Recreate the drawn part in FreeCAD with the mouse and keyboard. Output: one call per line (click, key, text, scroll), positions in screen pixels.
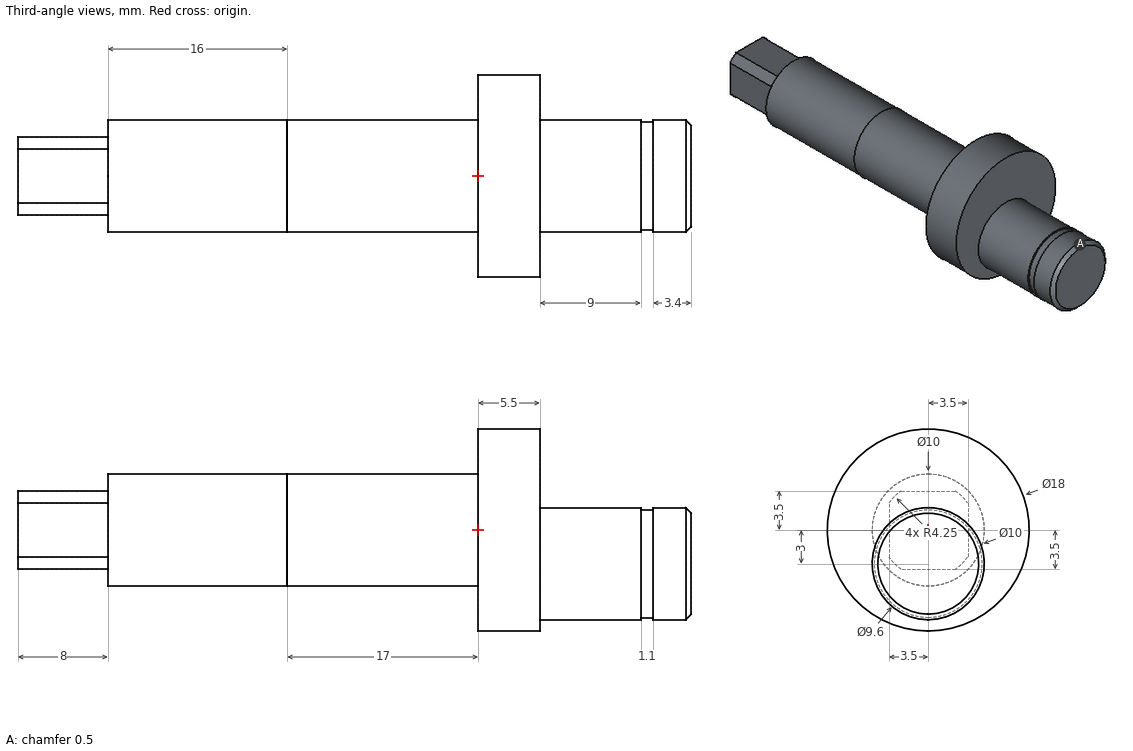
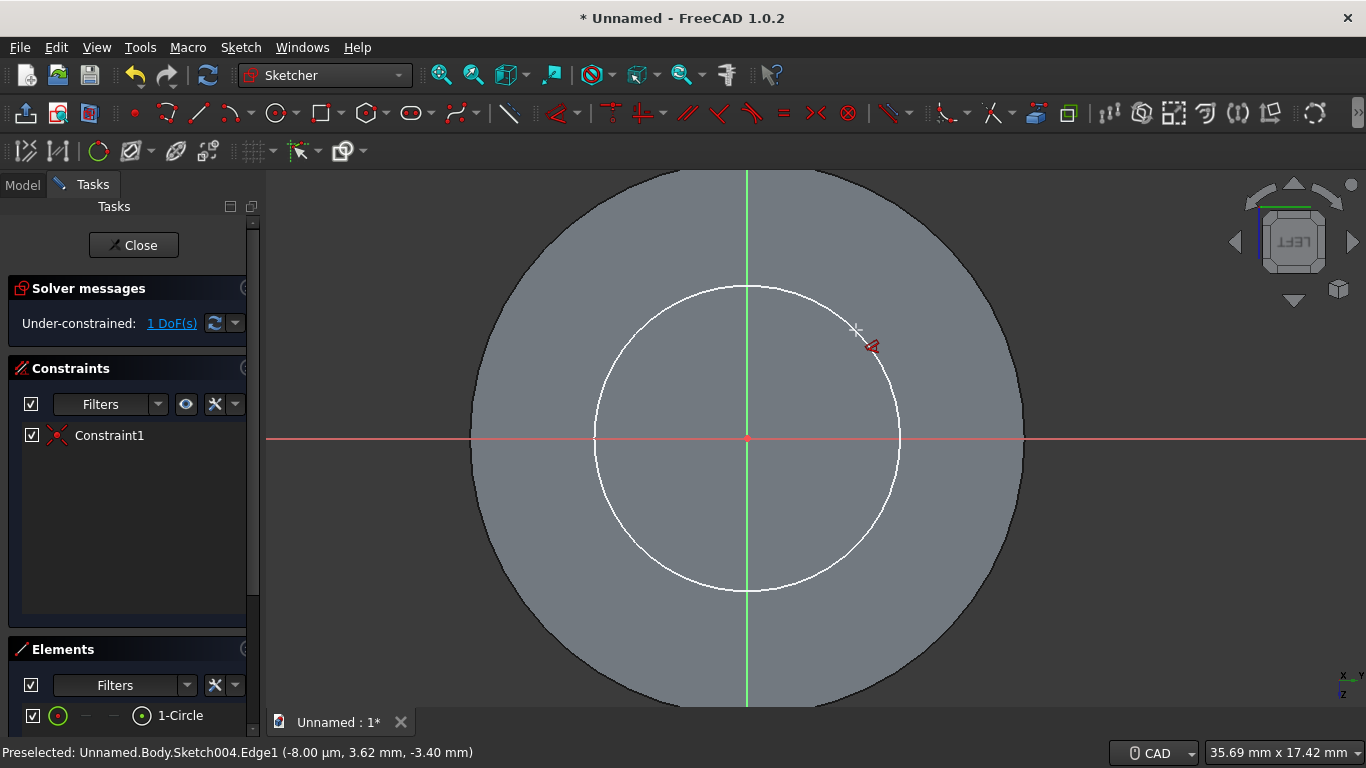
click(855, 330)
click(878, 307)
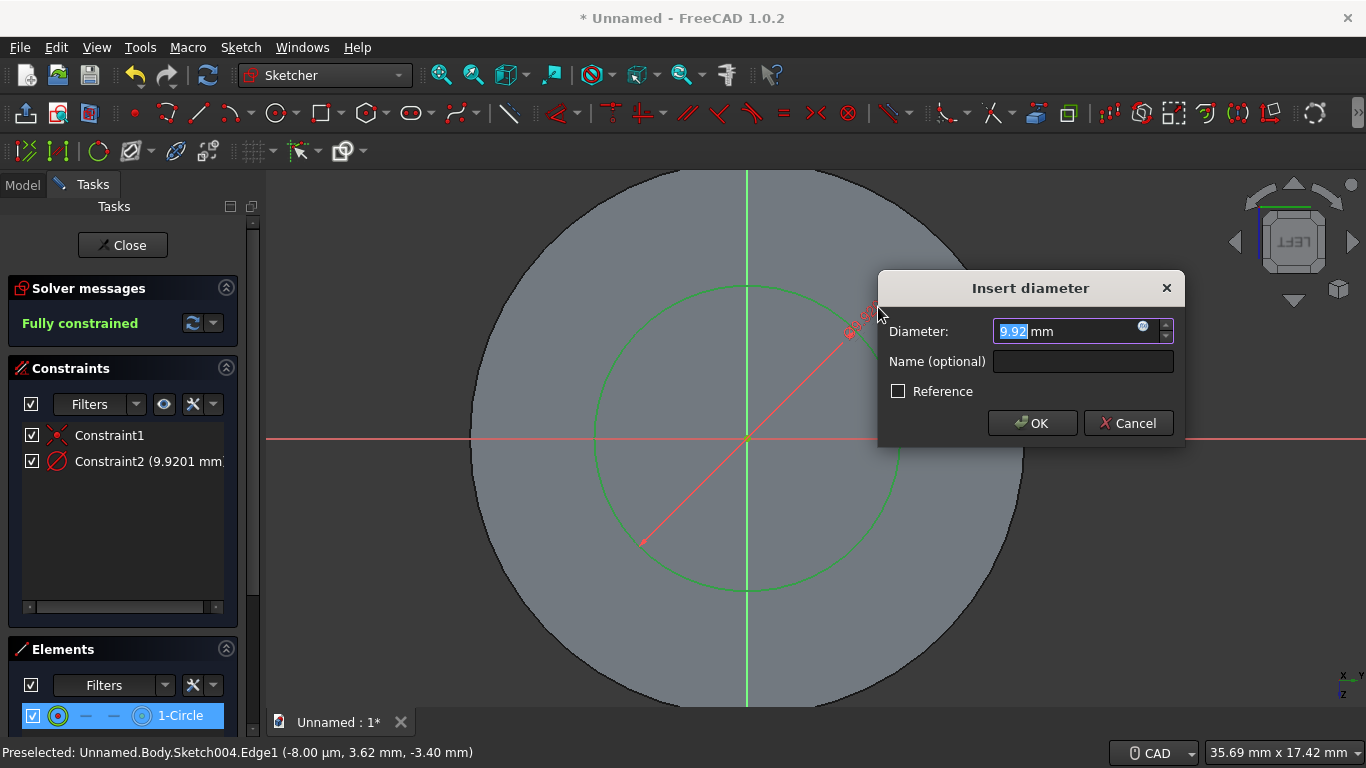
text(10)
key(Return)
key(Escape)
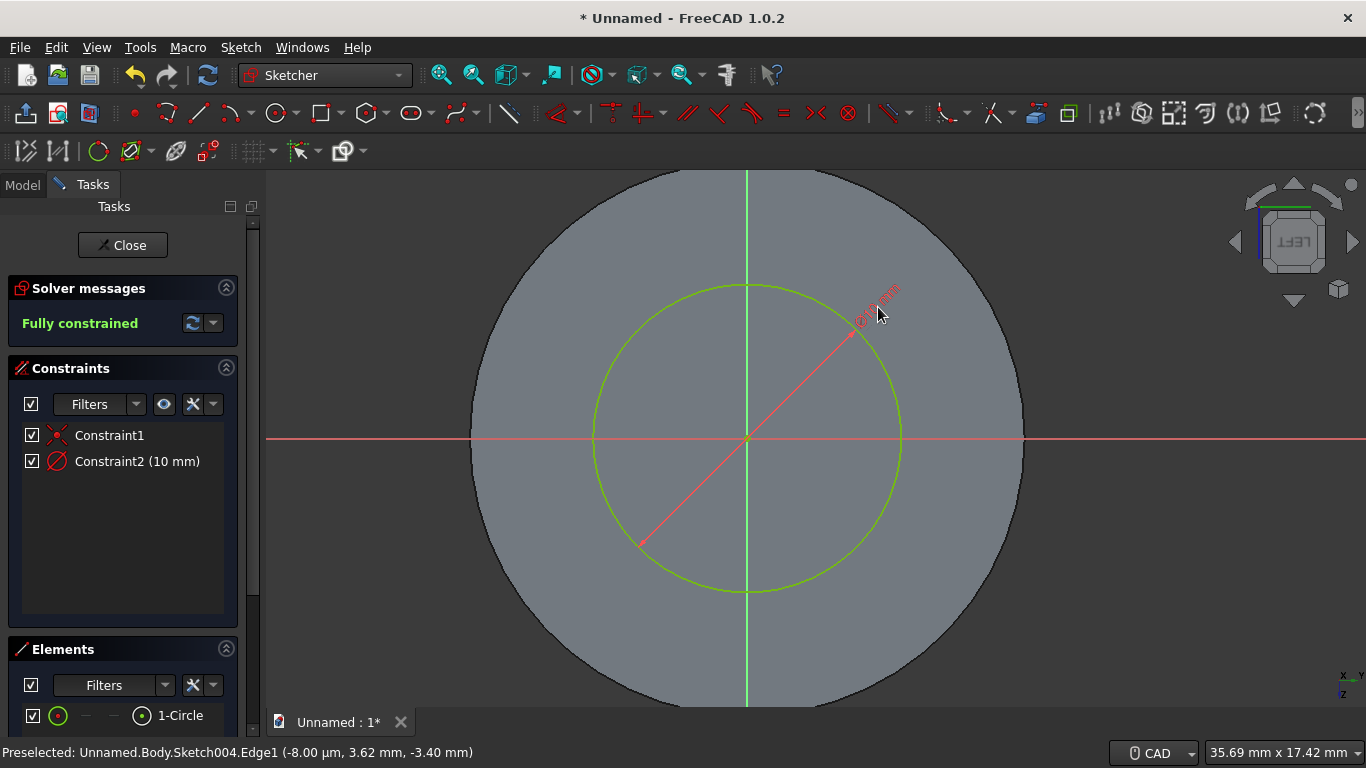
click(123, 245)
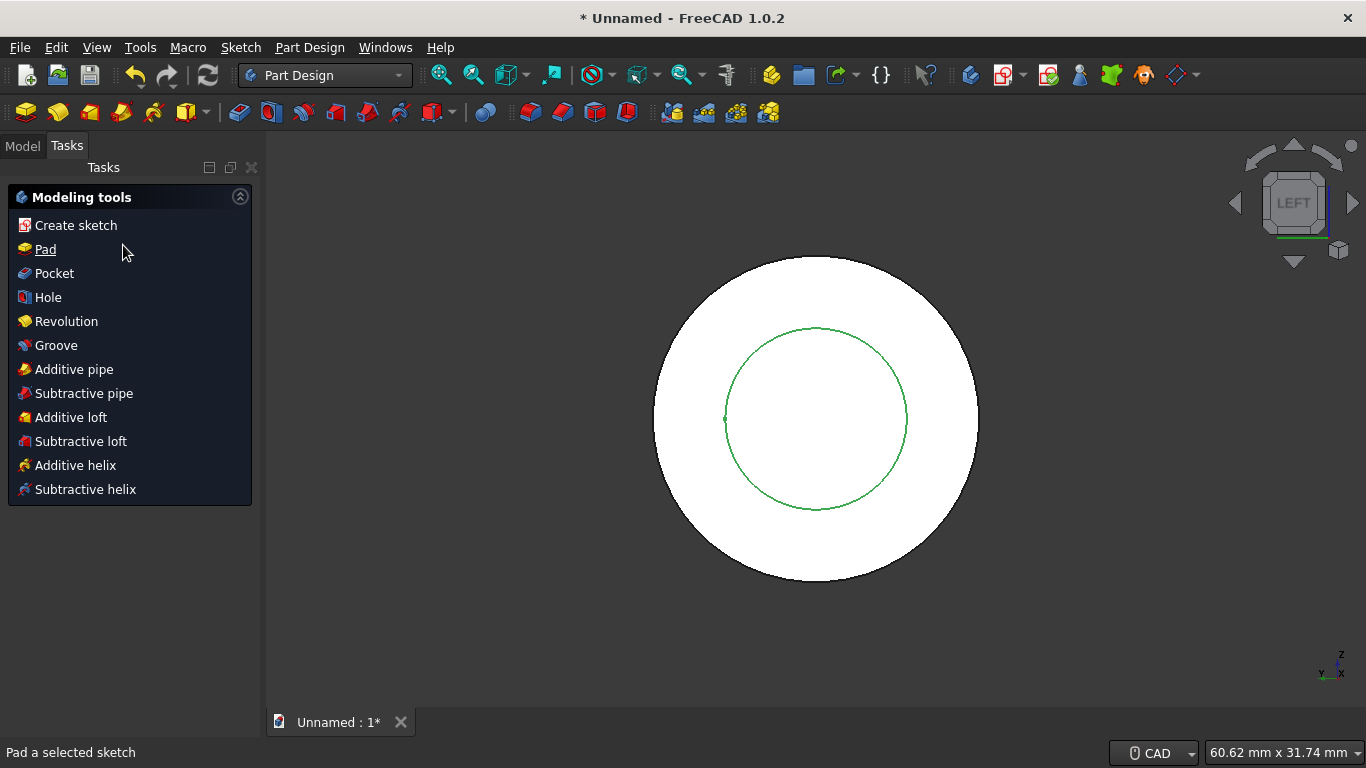
click(26, 112)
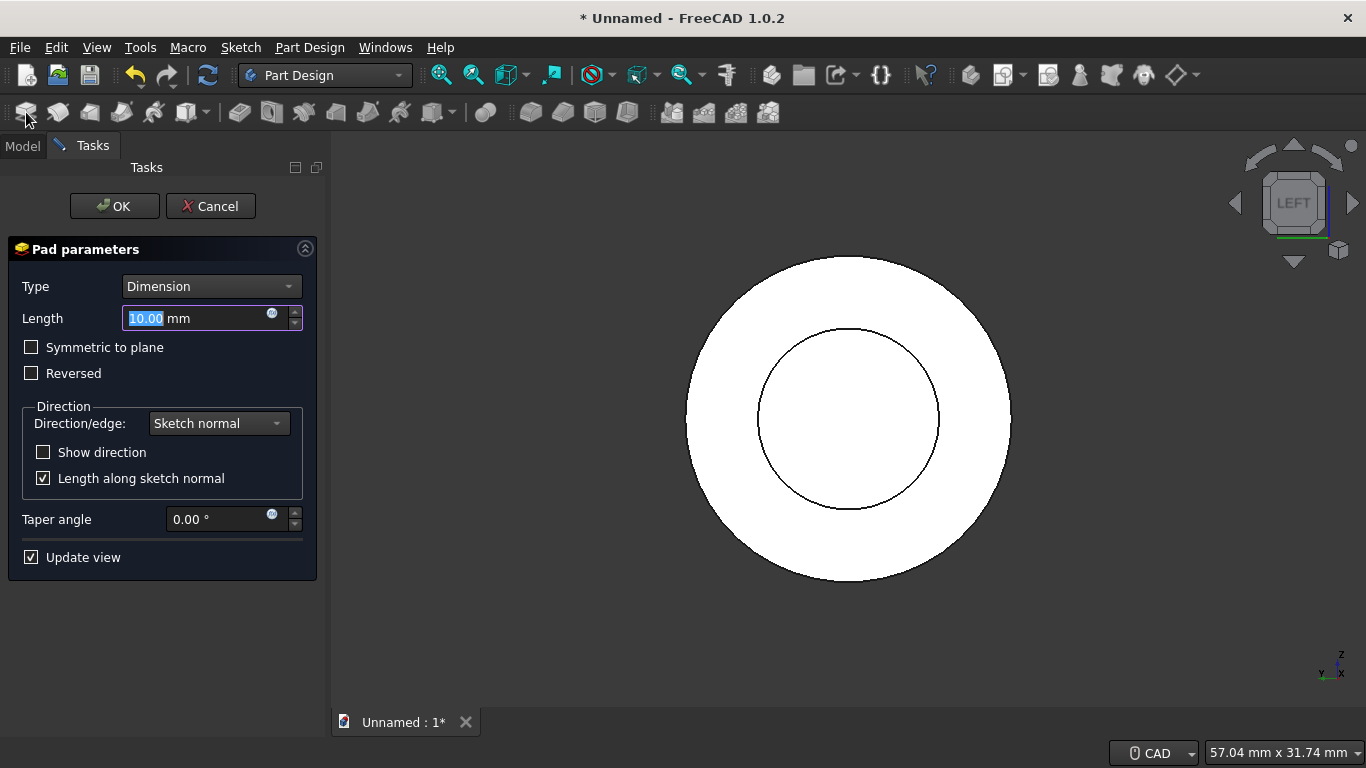
text(17)
key(Tab)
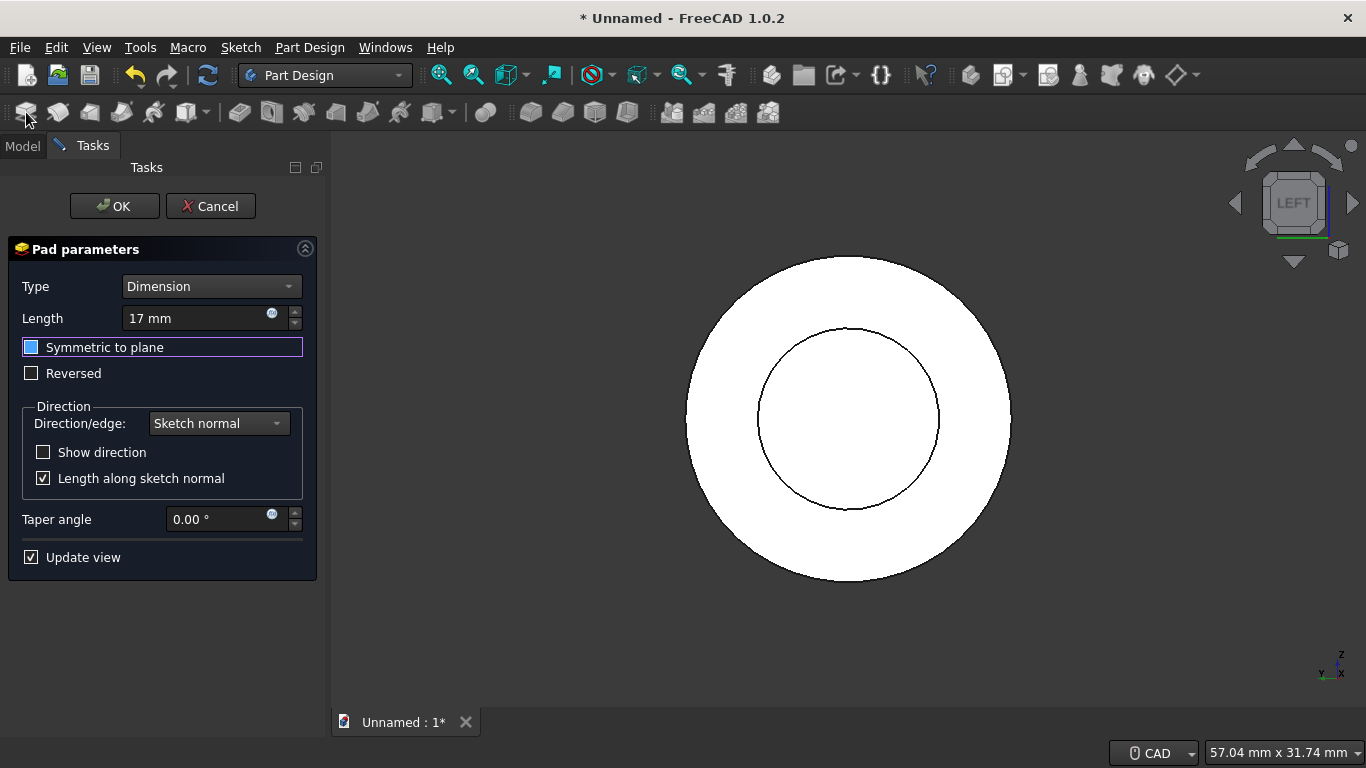
click(115, 206)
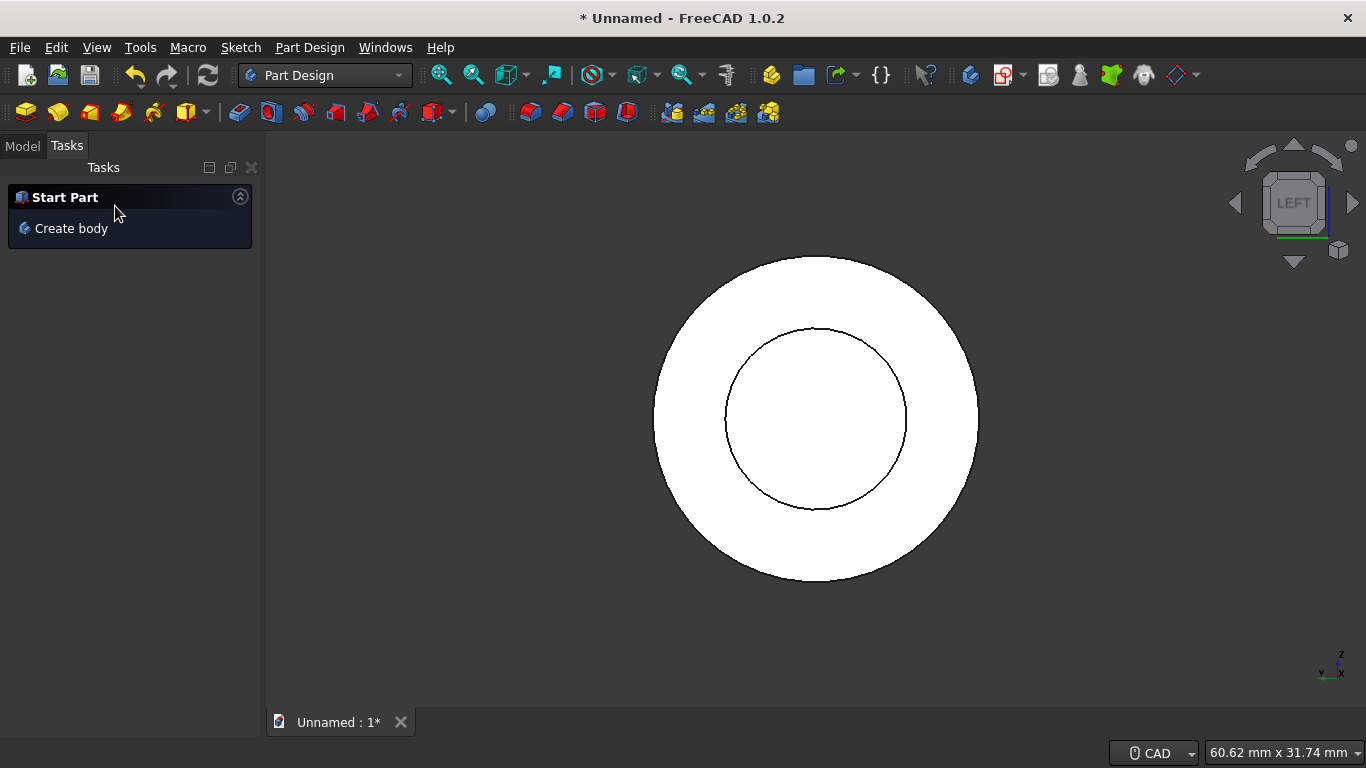
click(972, 76)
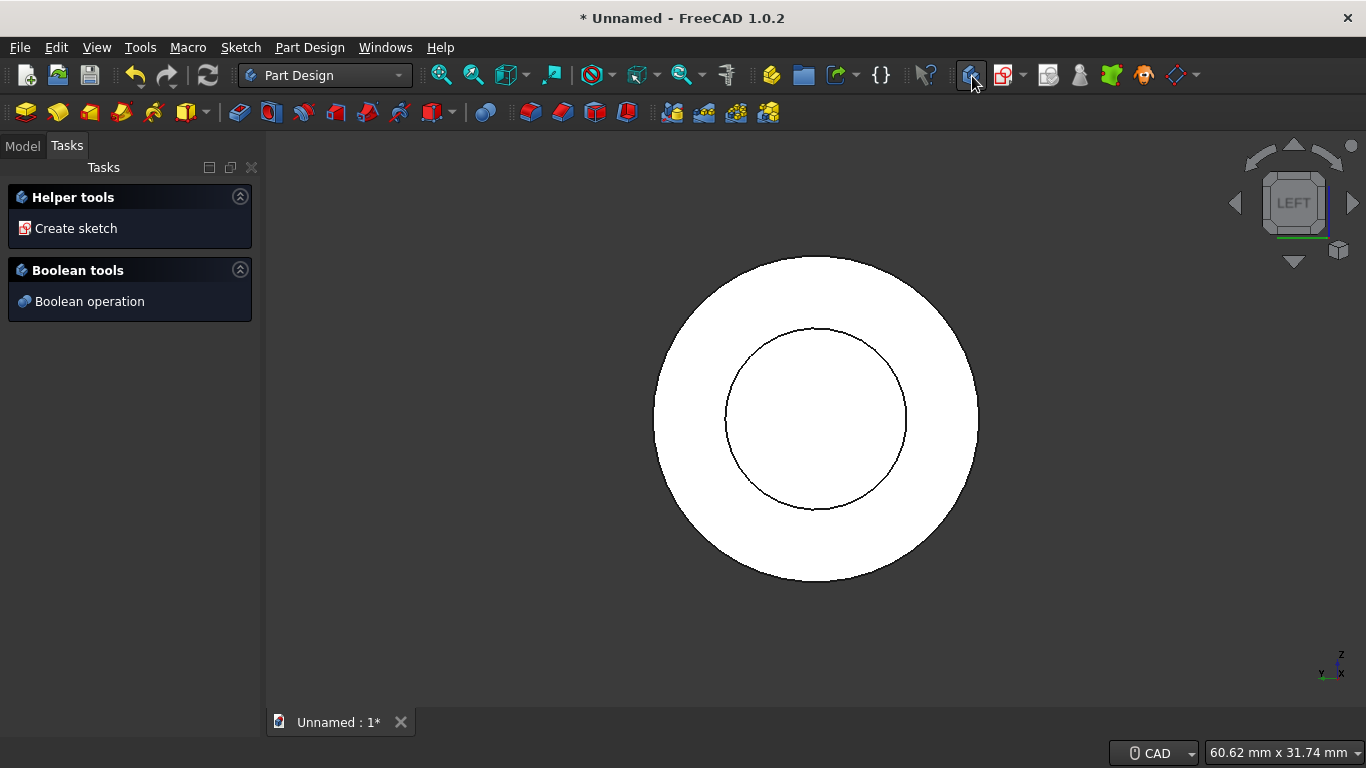
click(23, 145)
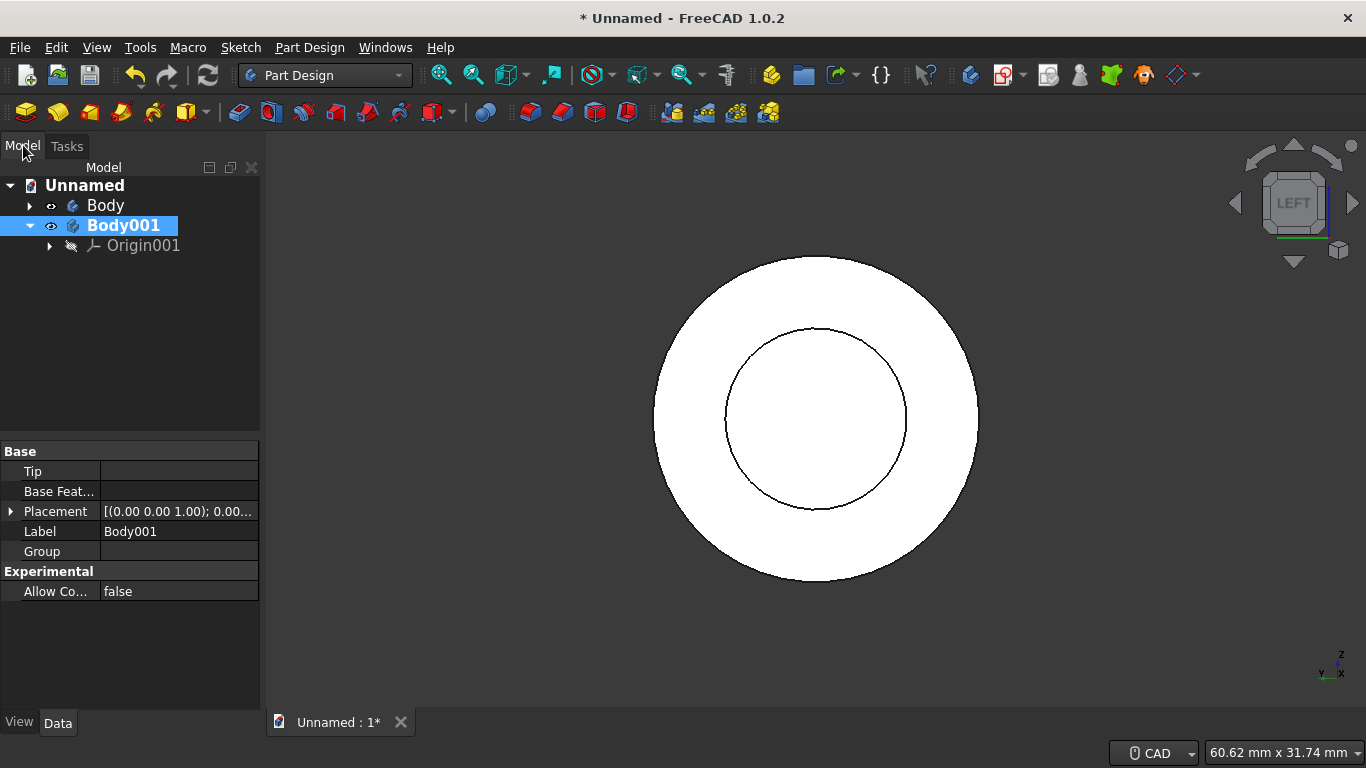
click(50, 246)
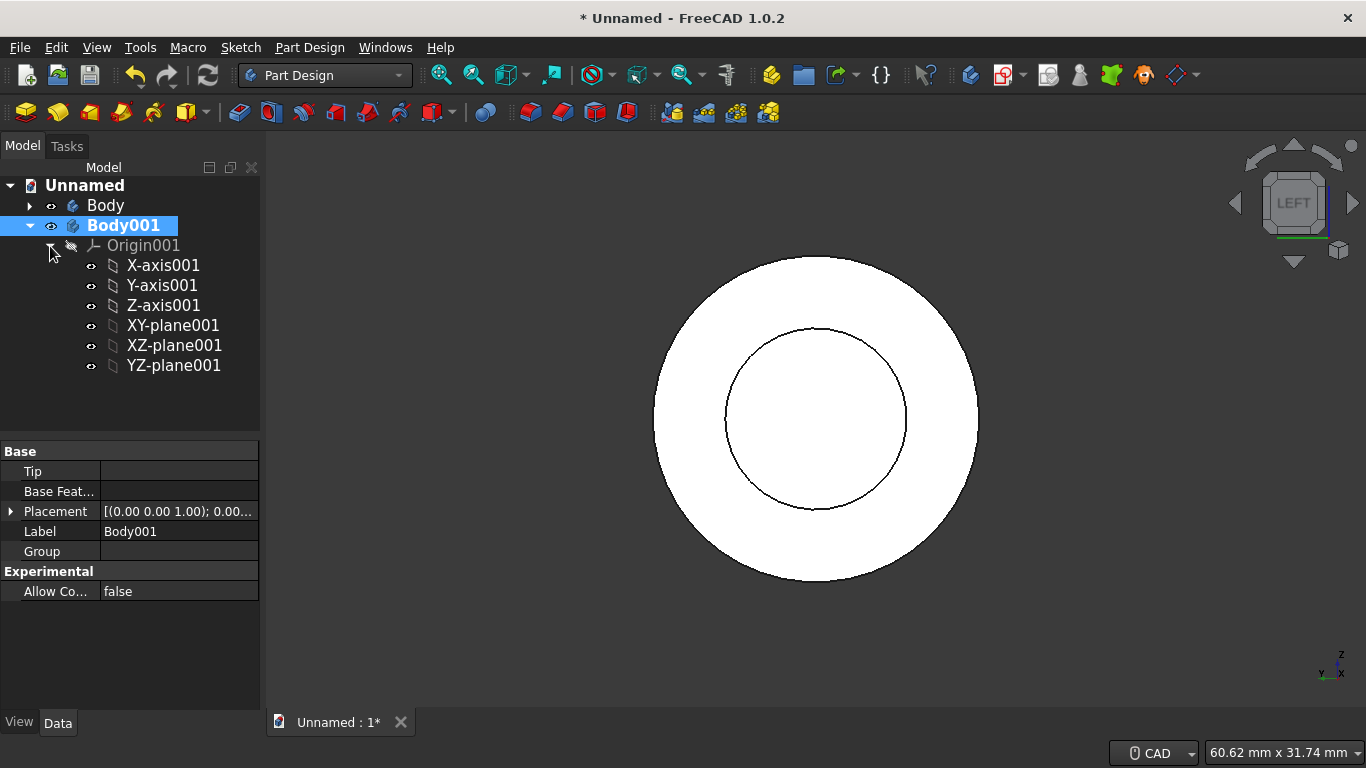
click(136, 366)